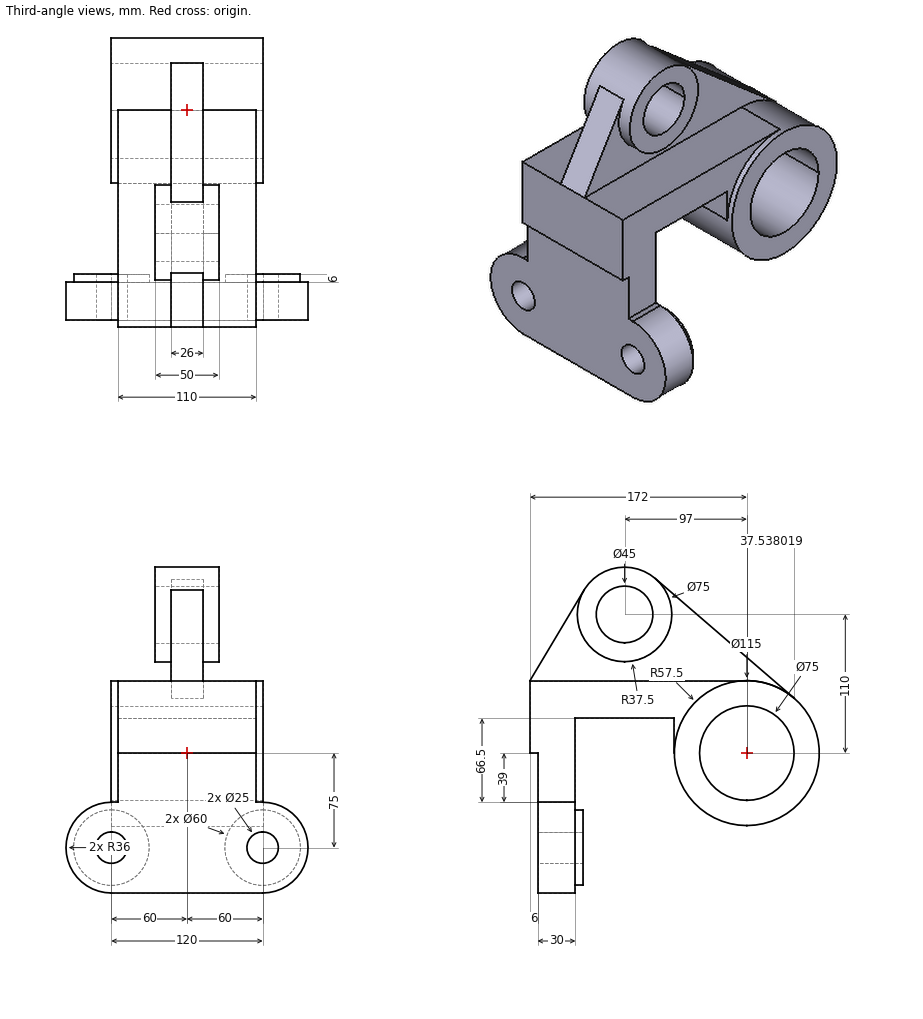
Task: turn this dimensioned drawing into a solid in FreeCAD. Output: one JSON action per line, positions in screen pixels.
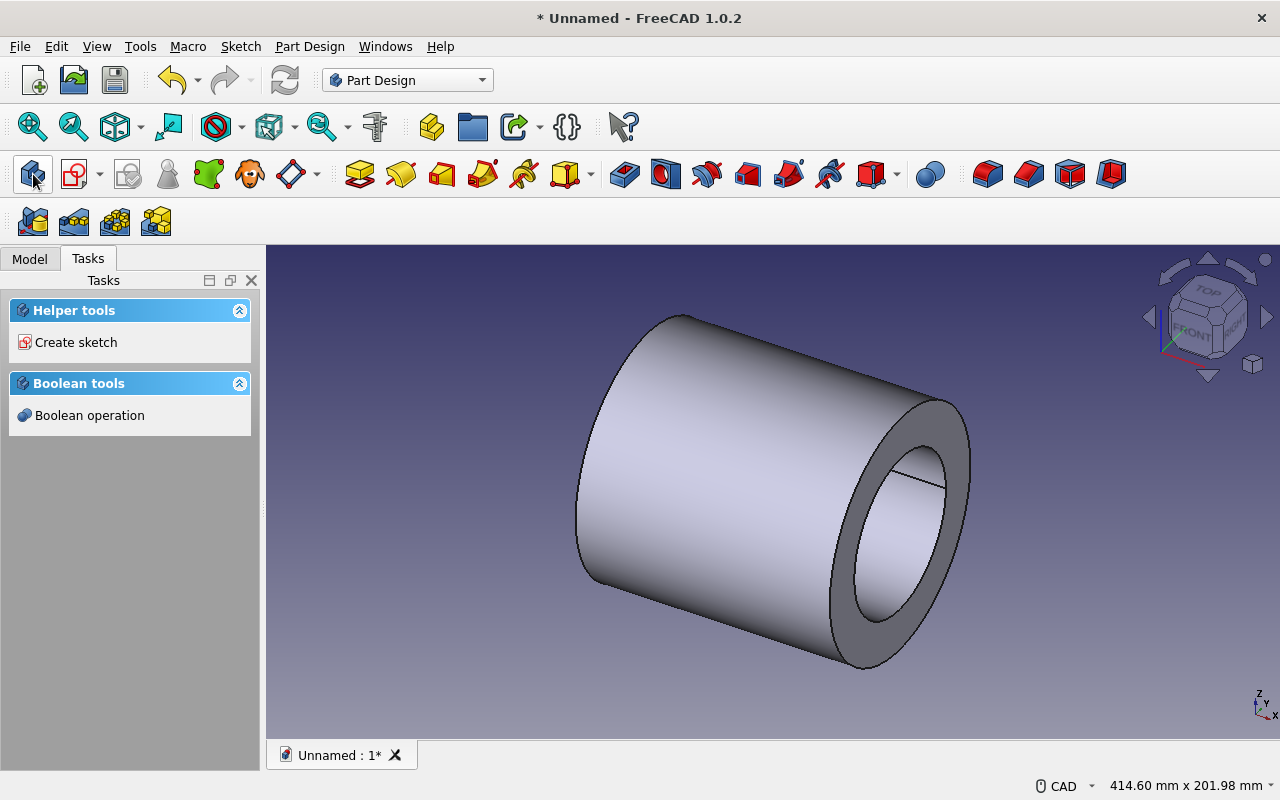
{"action": "left_click", "coordinate": [30, 258]}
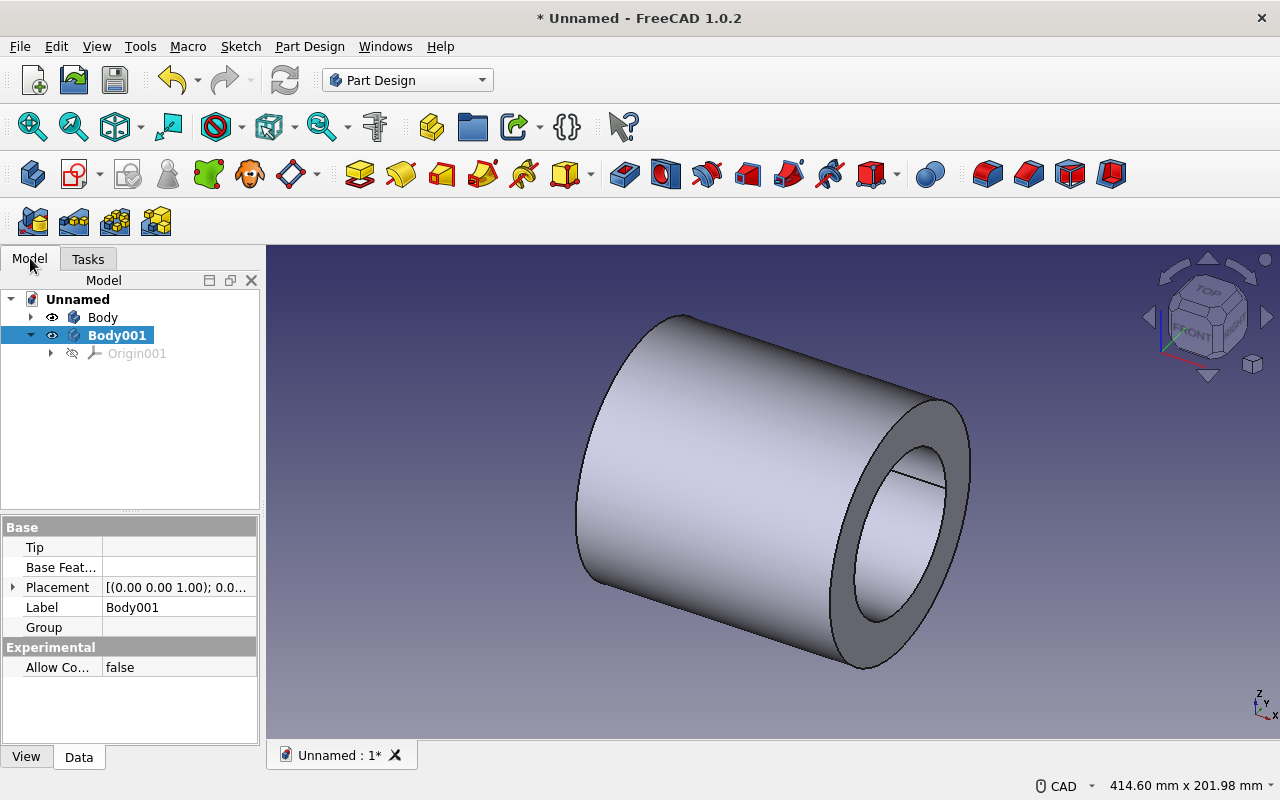
{"action": "left_click", "coordinate": [51, 353]}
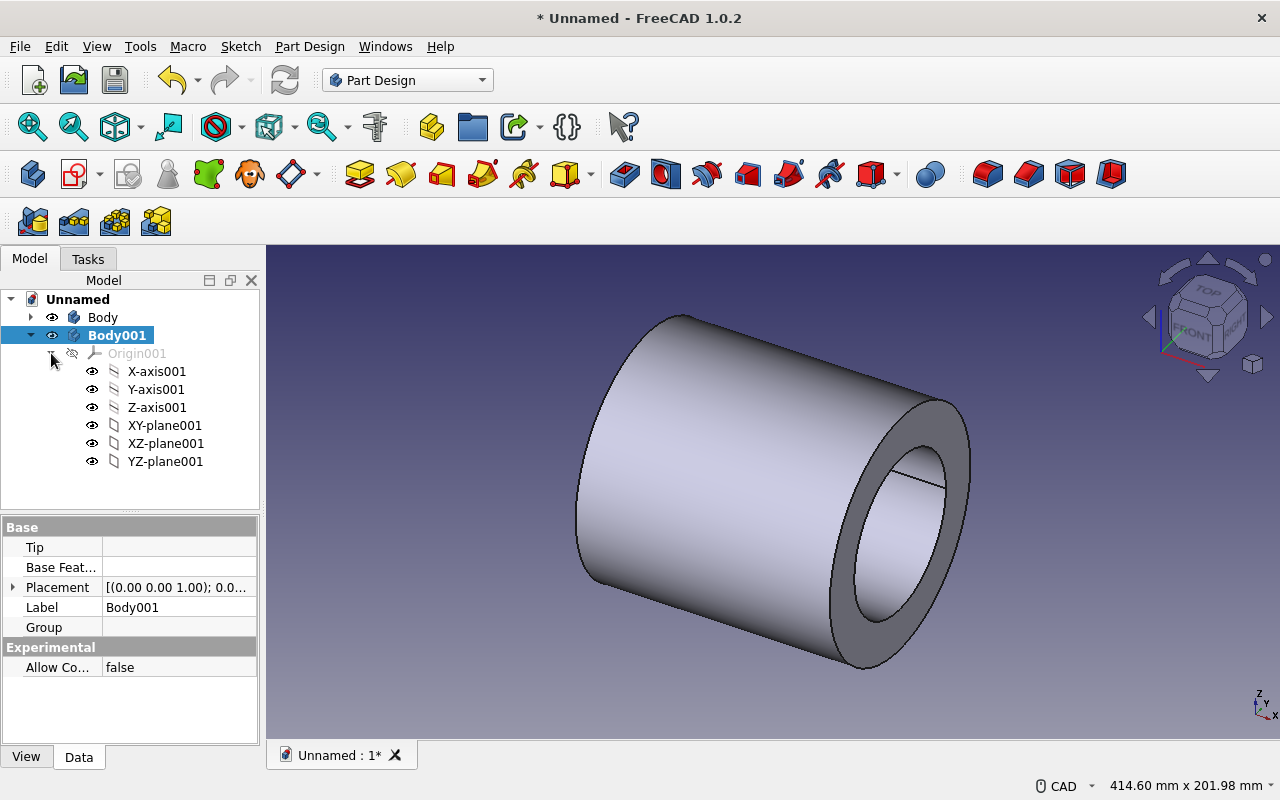
{"action": "left_click", "coordinate": [137, 443]}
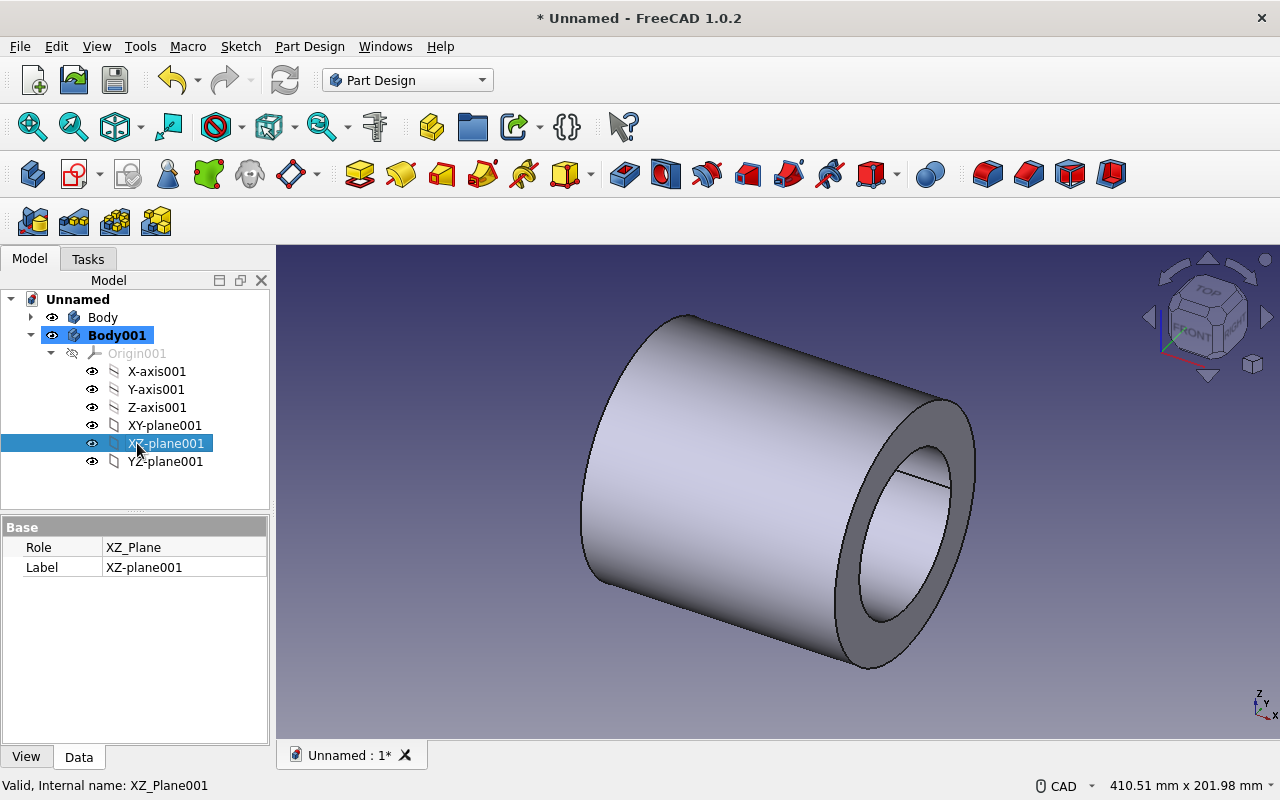
{"action": "left_click", "coordinate": [290, 174]}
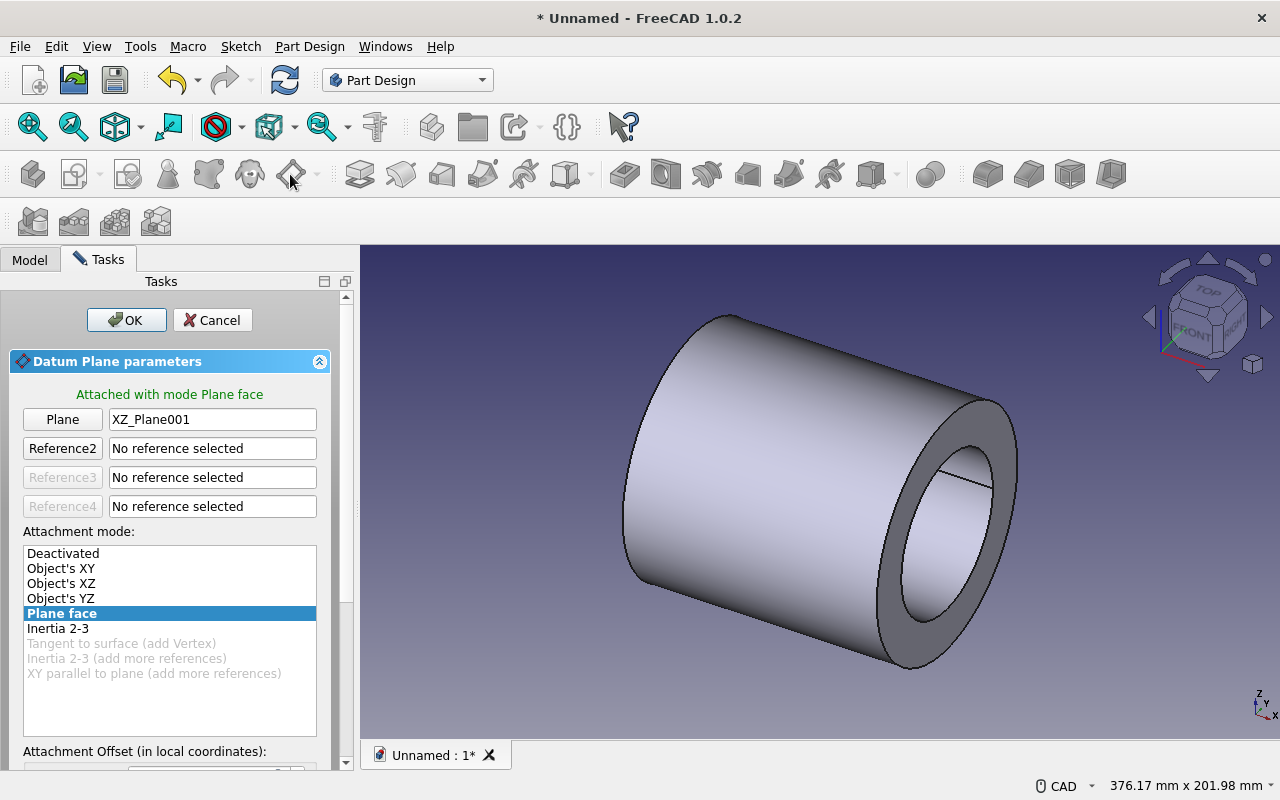
{"action": "scroll", "coordinate": [346, 530], "scroll_direction": "down", "scroll_amount": 3}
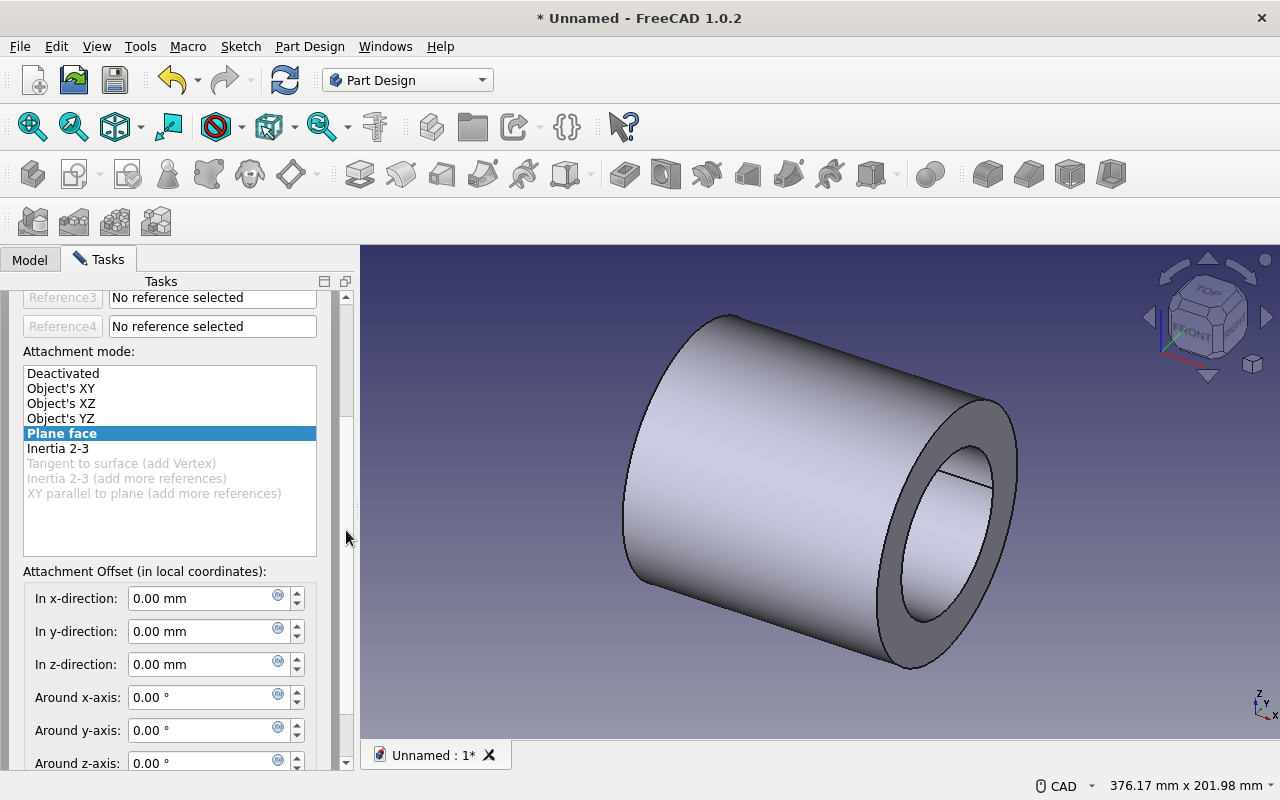
{"action": "triple_click", "coordinate": [210, 664]}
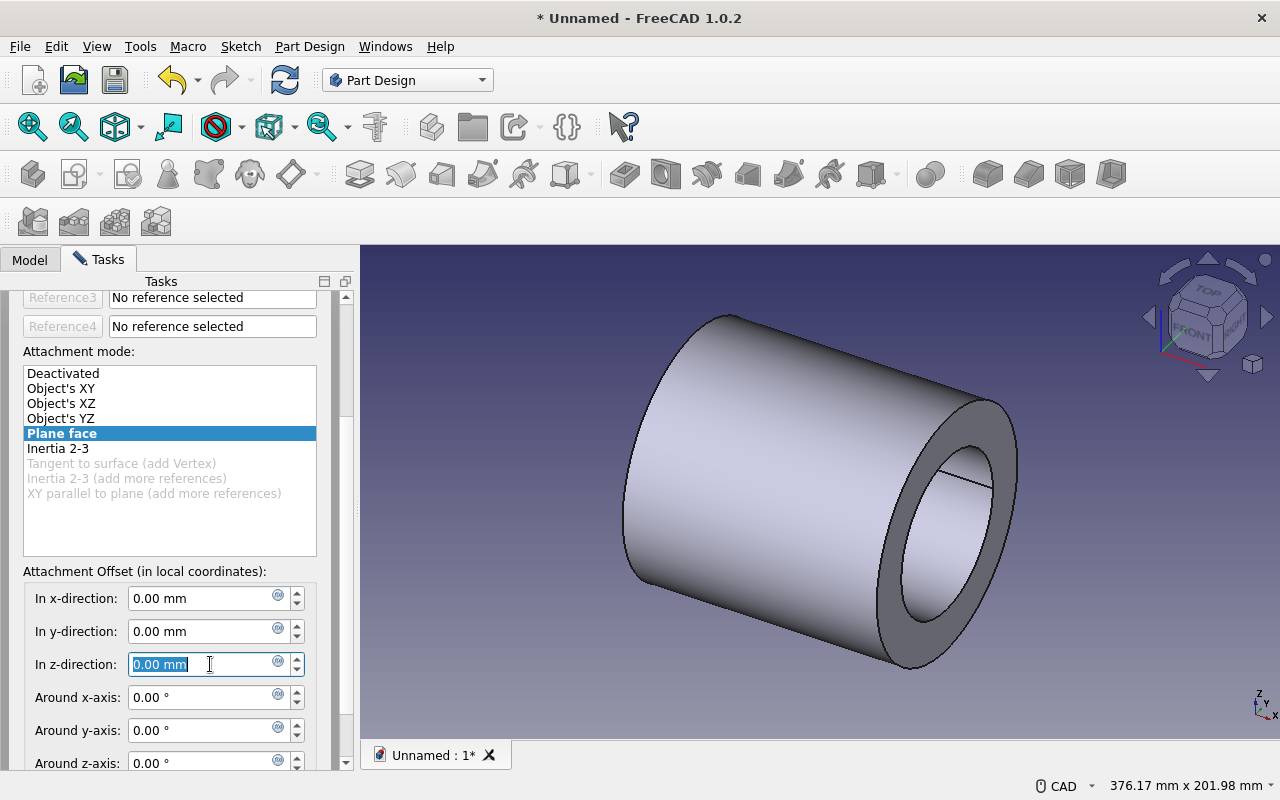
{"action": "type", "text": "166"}
{"action": "key", "text": "Tab"}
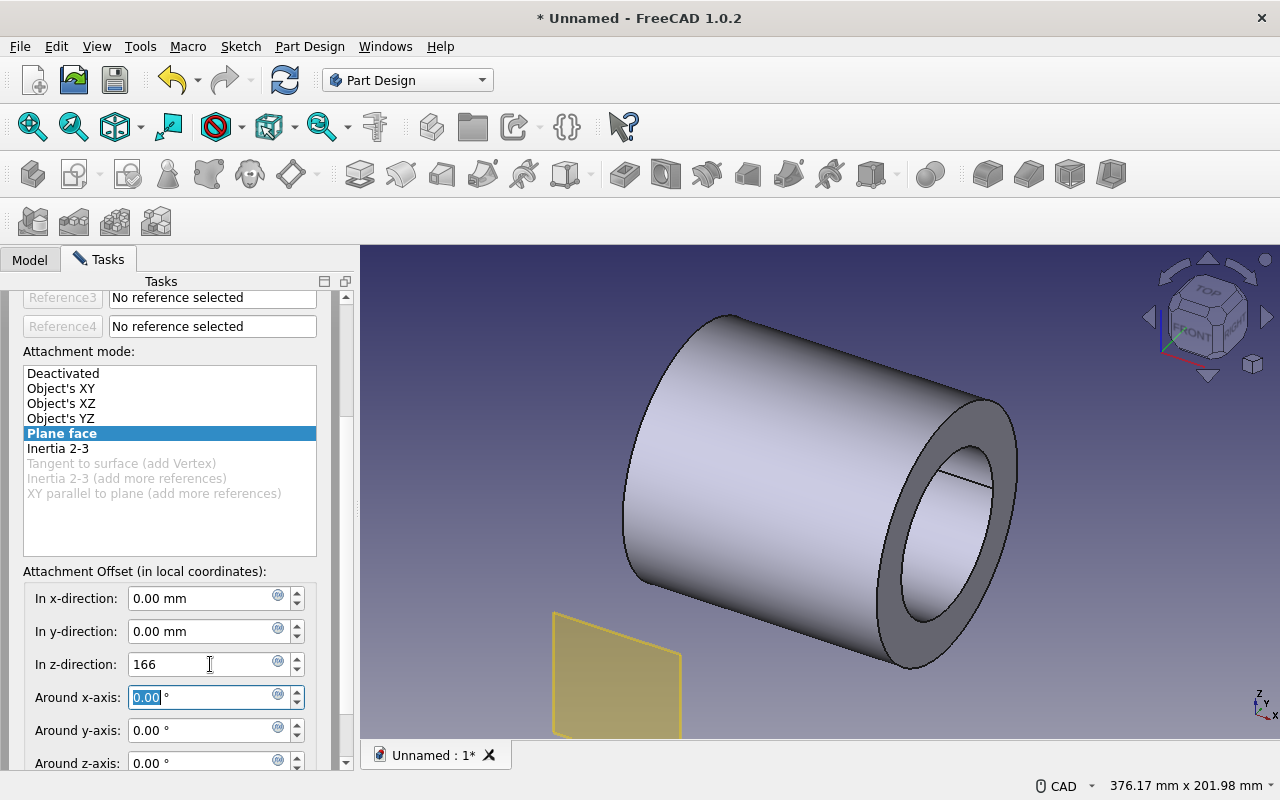
{"action": "scroll", "coordinate": [346, 530], "scroll_direction": "up", "scroll_amount": 4}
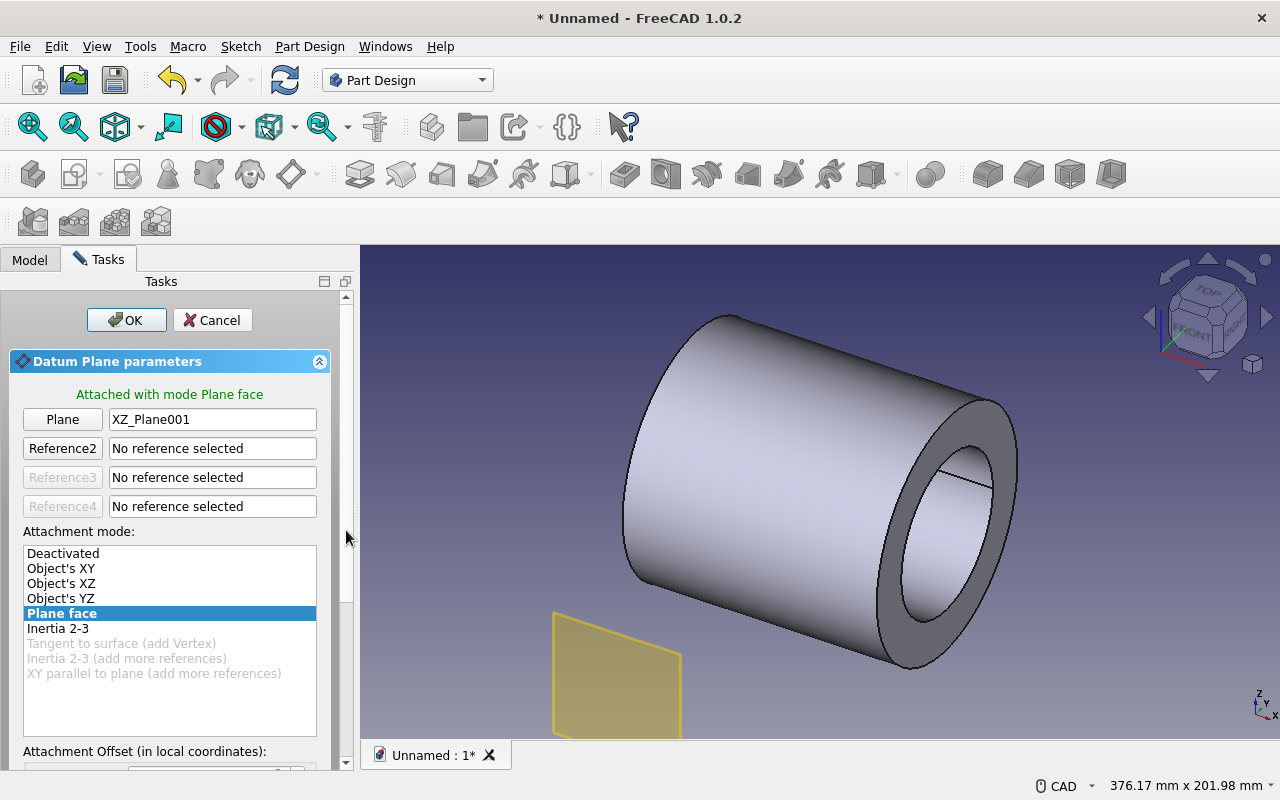
{"action": "left_click", "coordinate": [127, 320]}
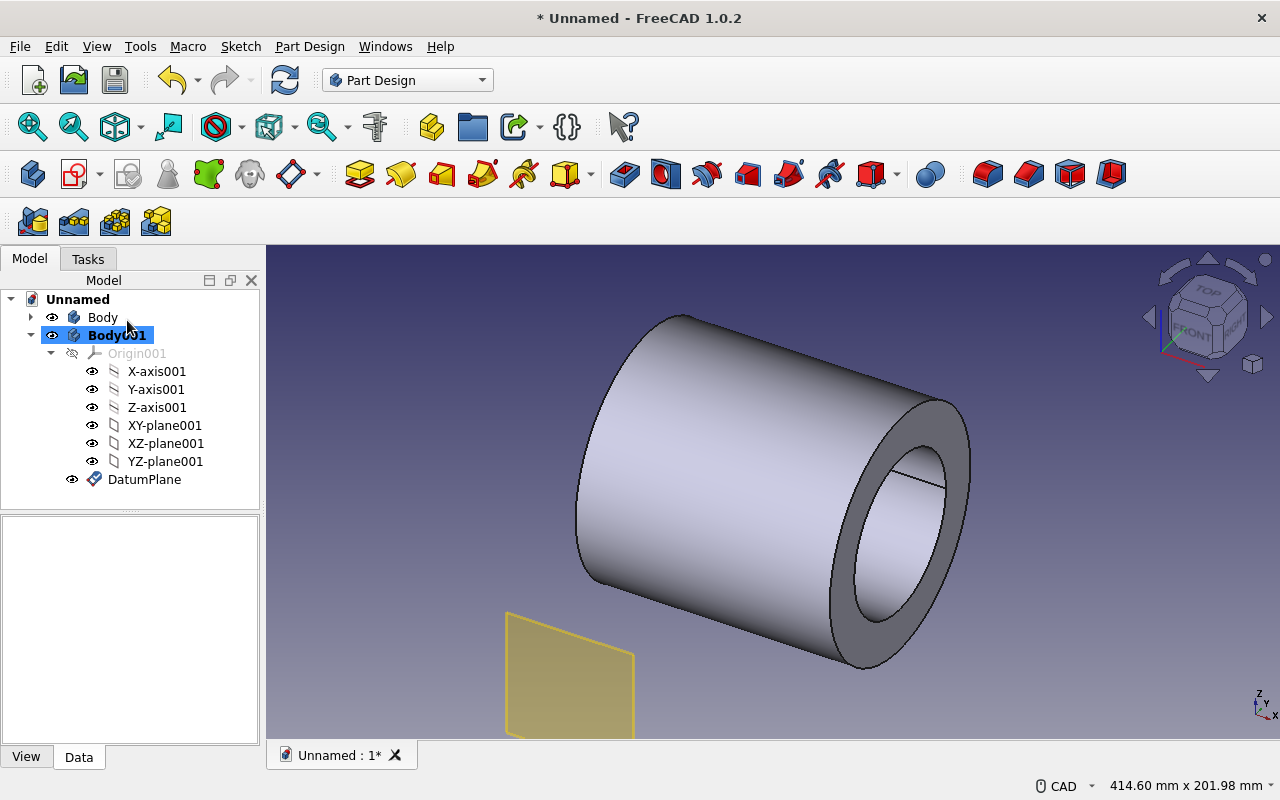
{"action": "left_click", "coordinate": [117, 479]}